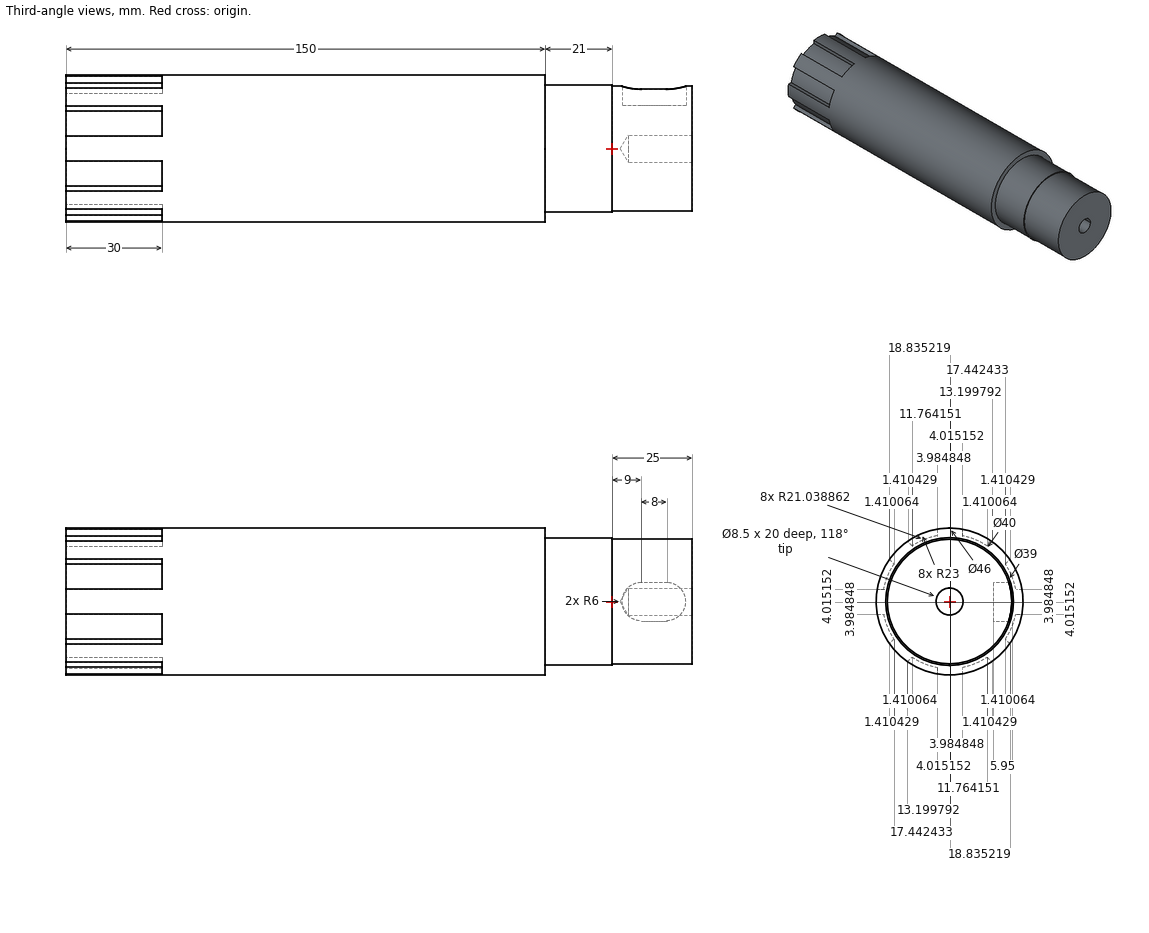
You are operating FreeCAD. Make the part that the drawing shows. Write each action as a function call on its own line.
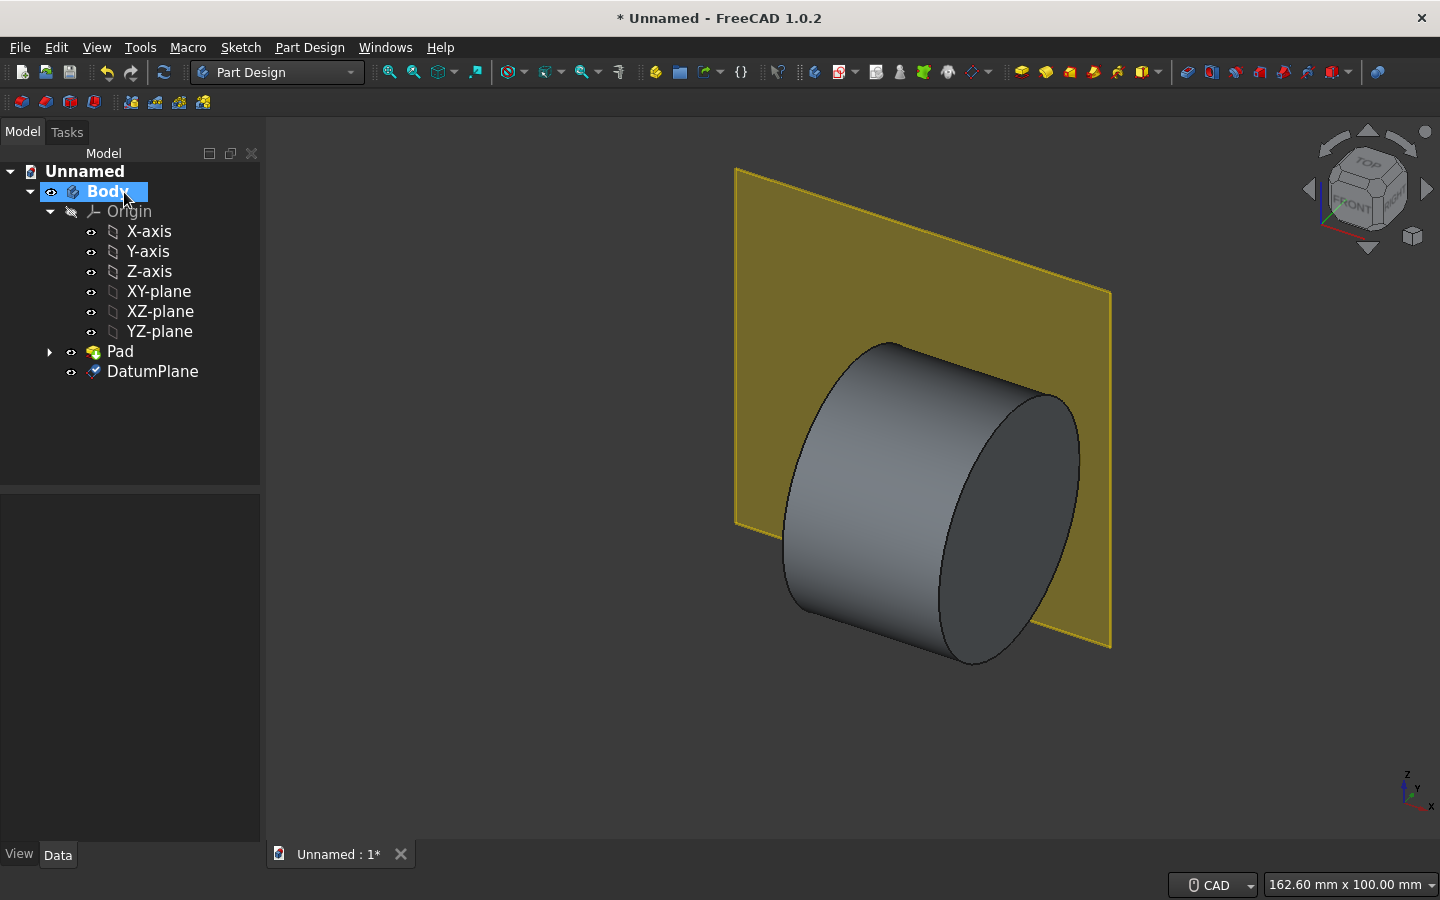
click(116, 372)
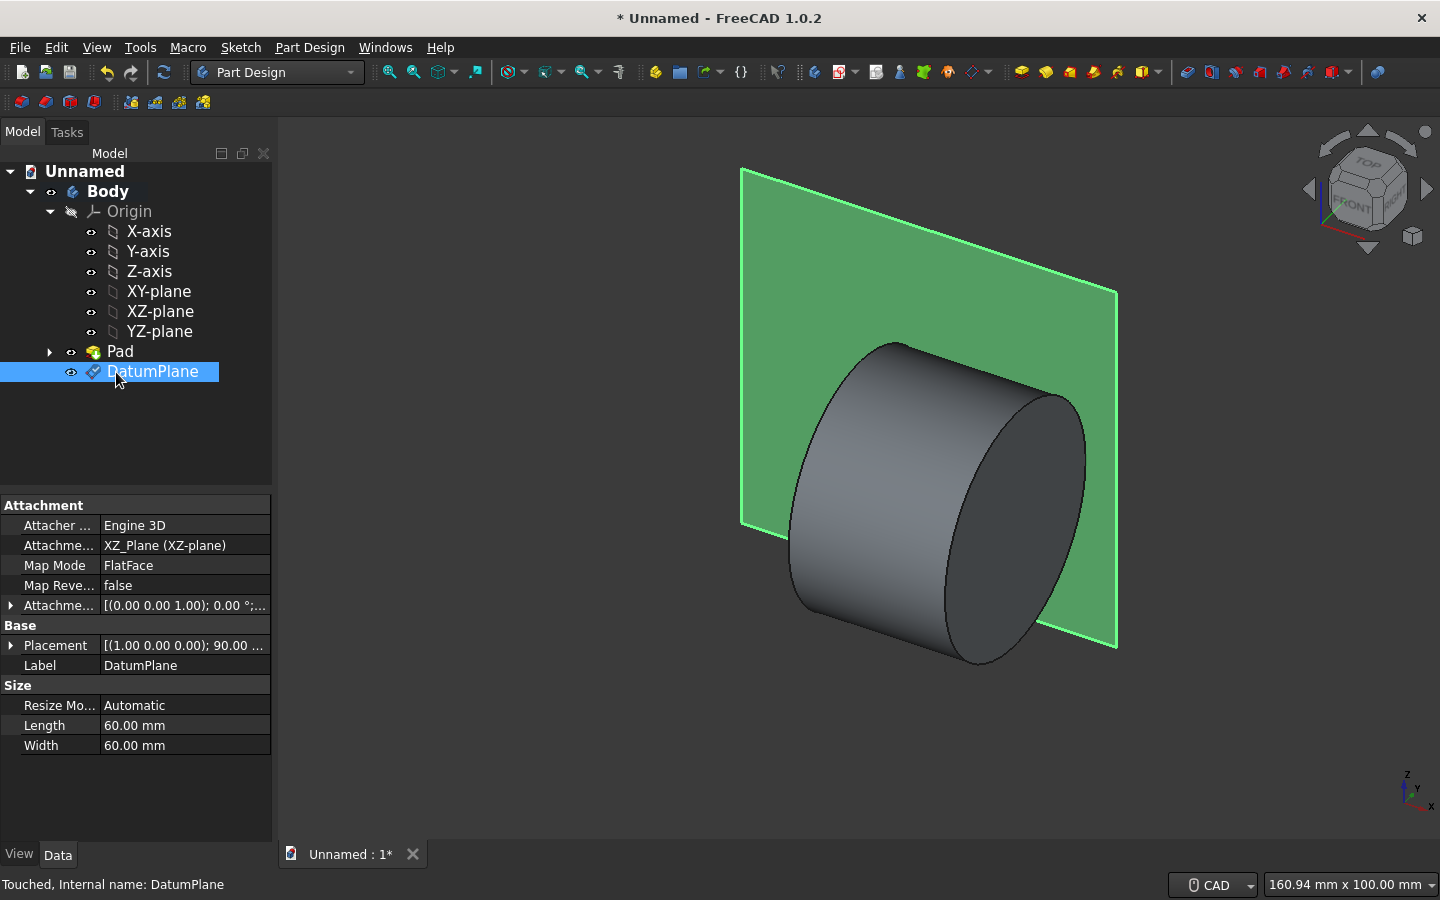
click(840, 72)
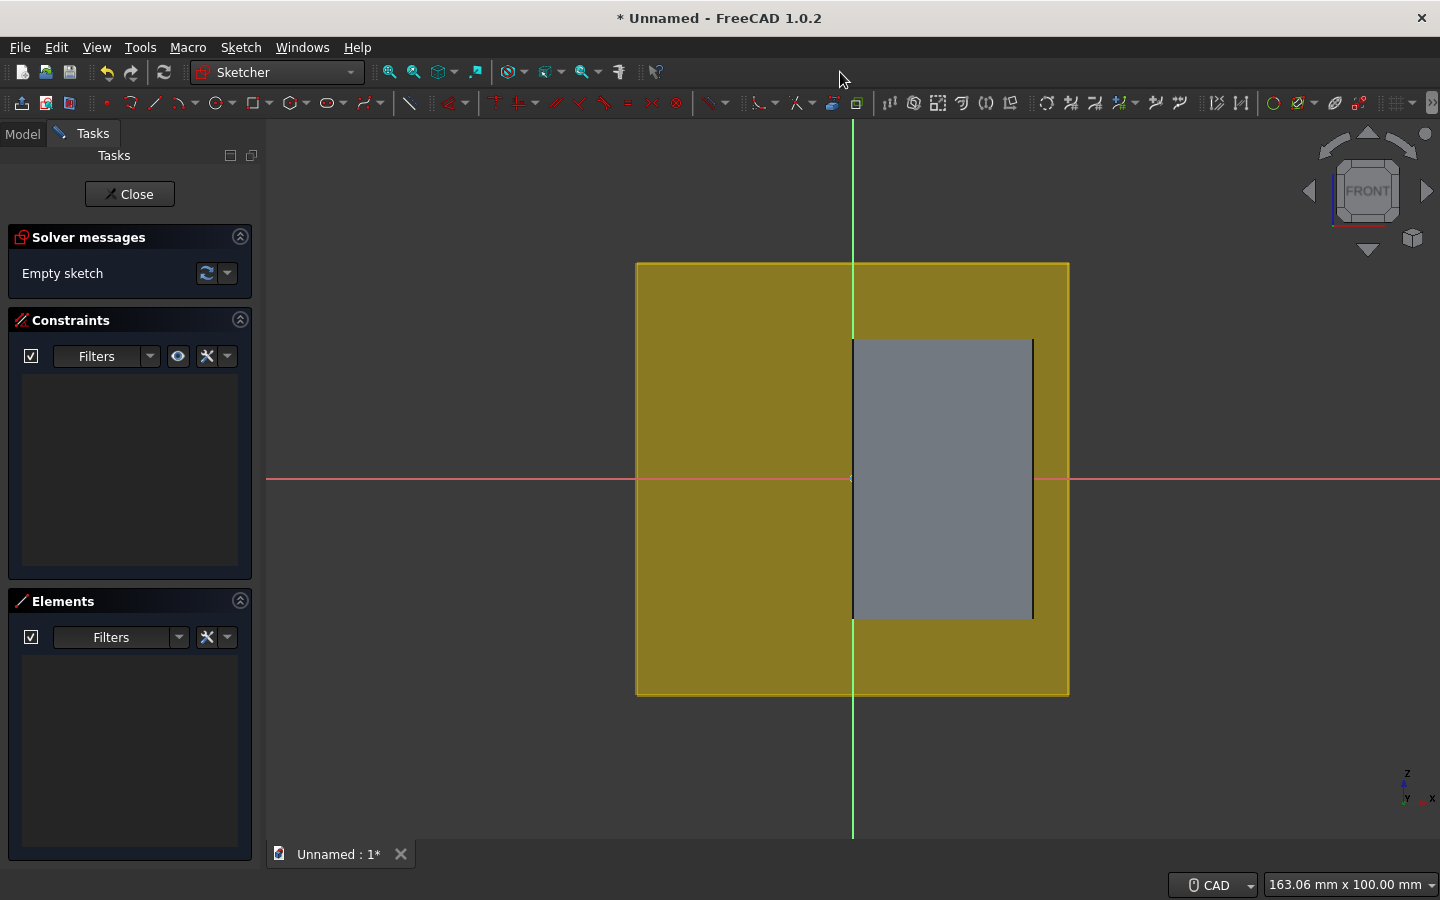
click(70, 104)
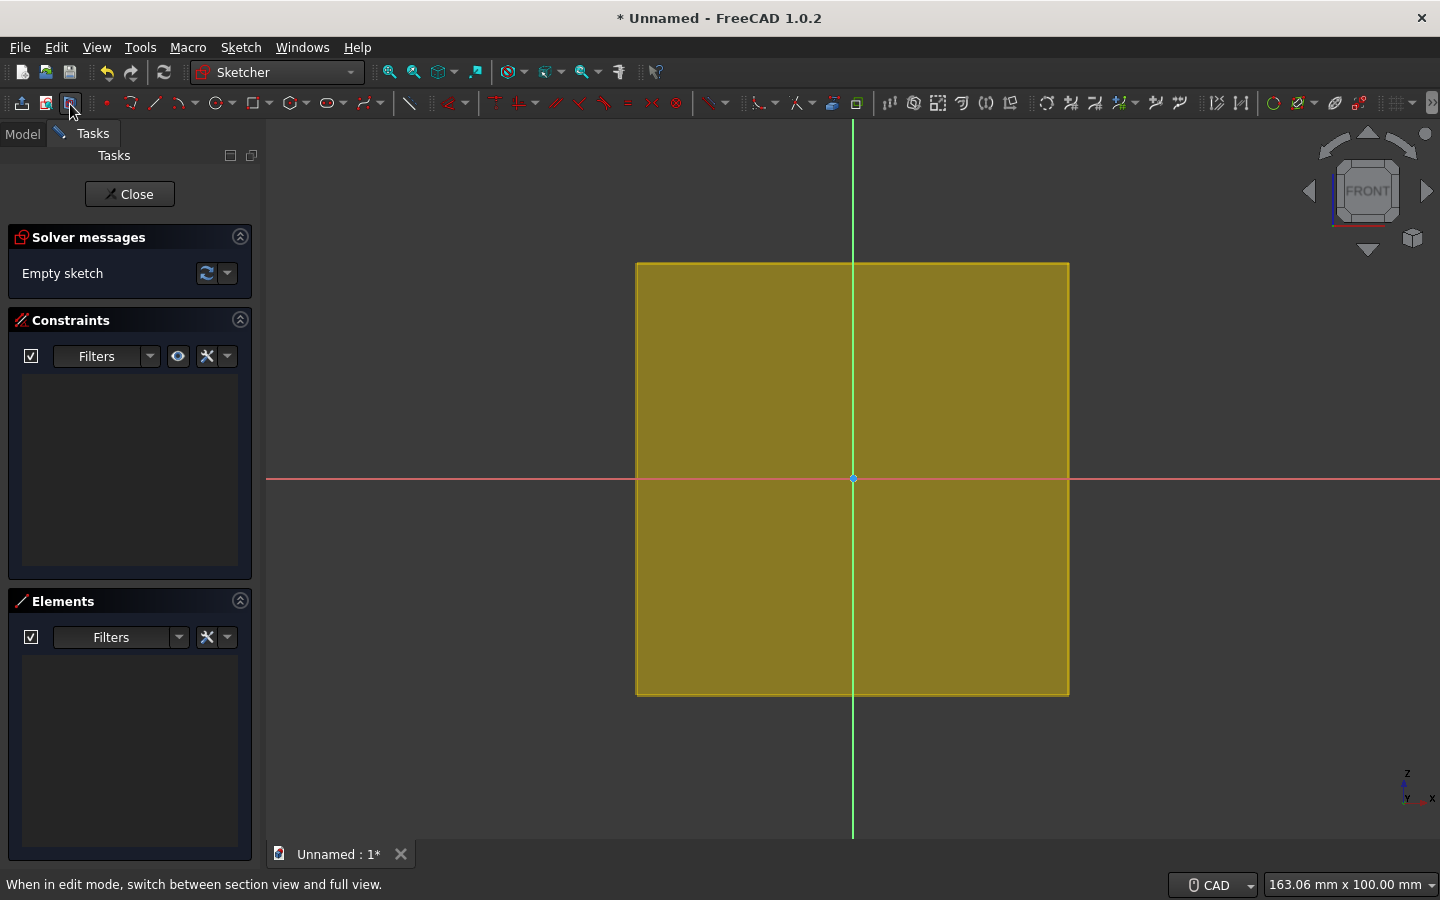
scroll(985, 479, up, 7)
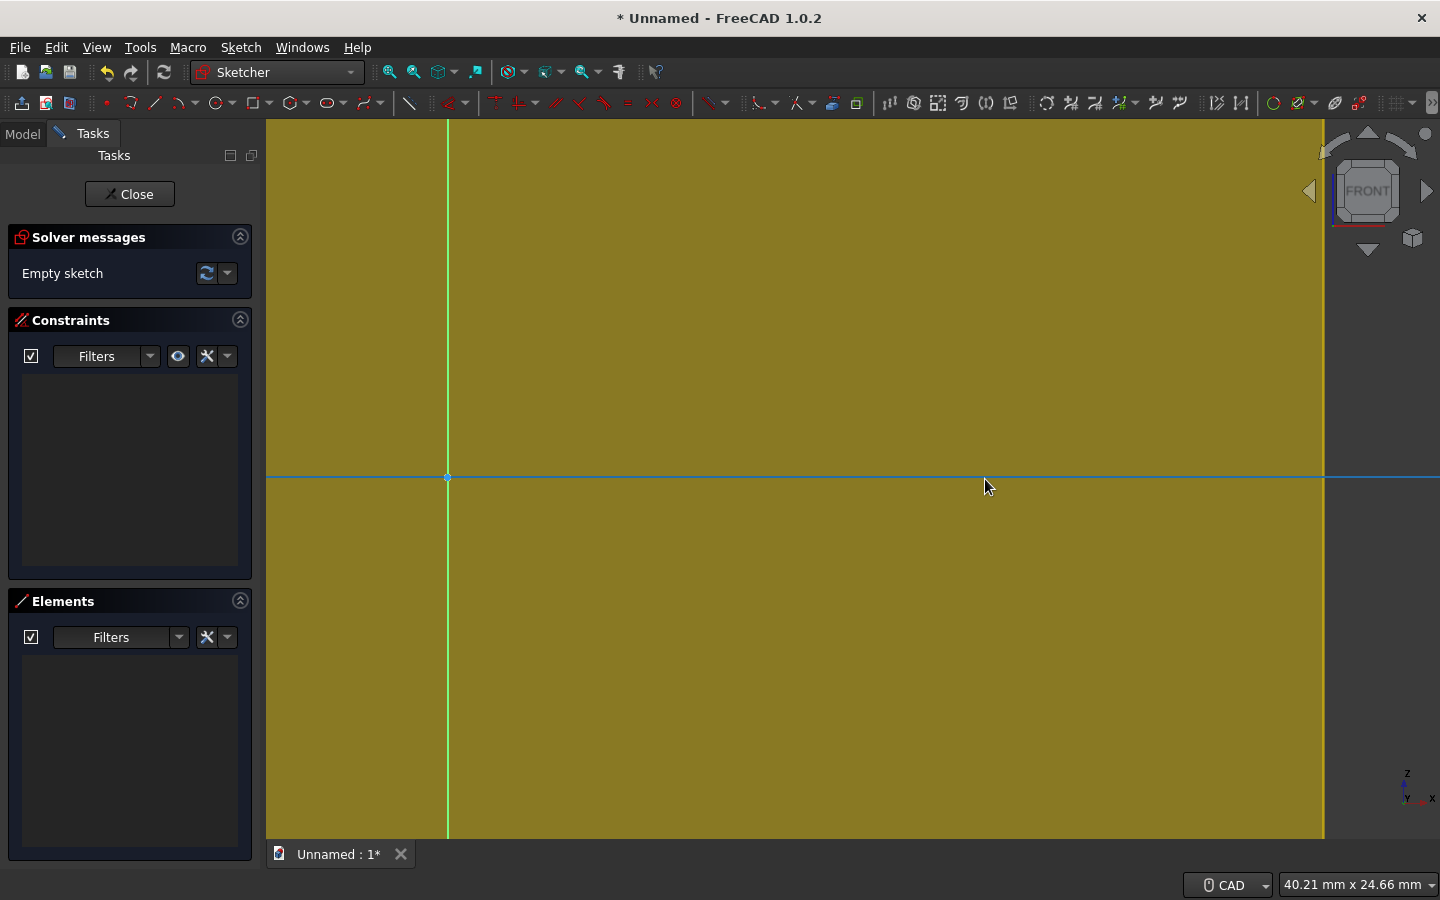
click(328, 104)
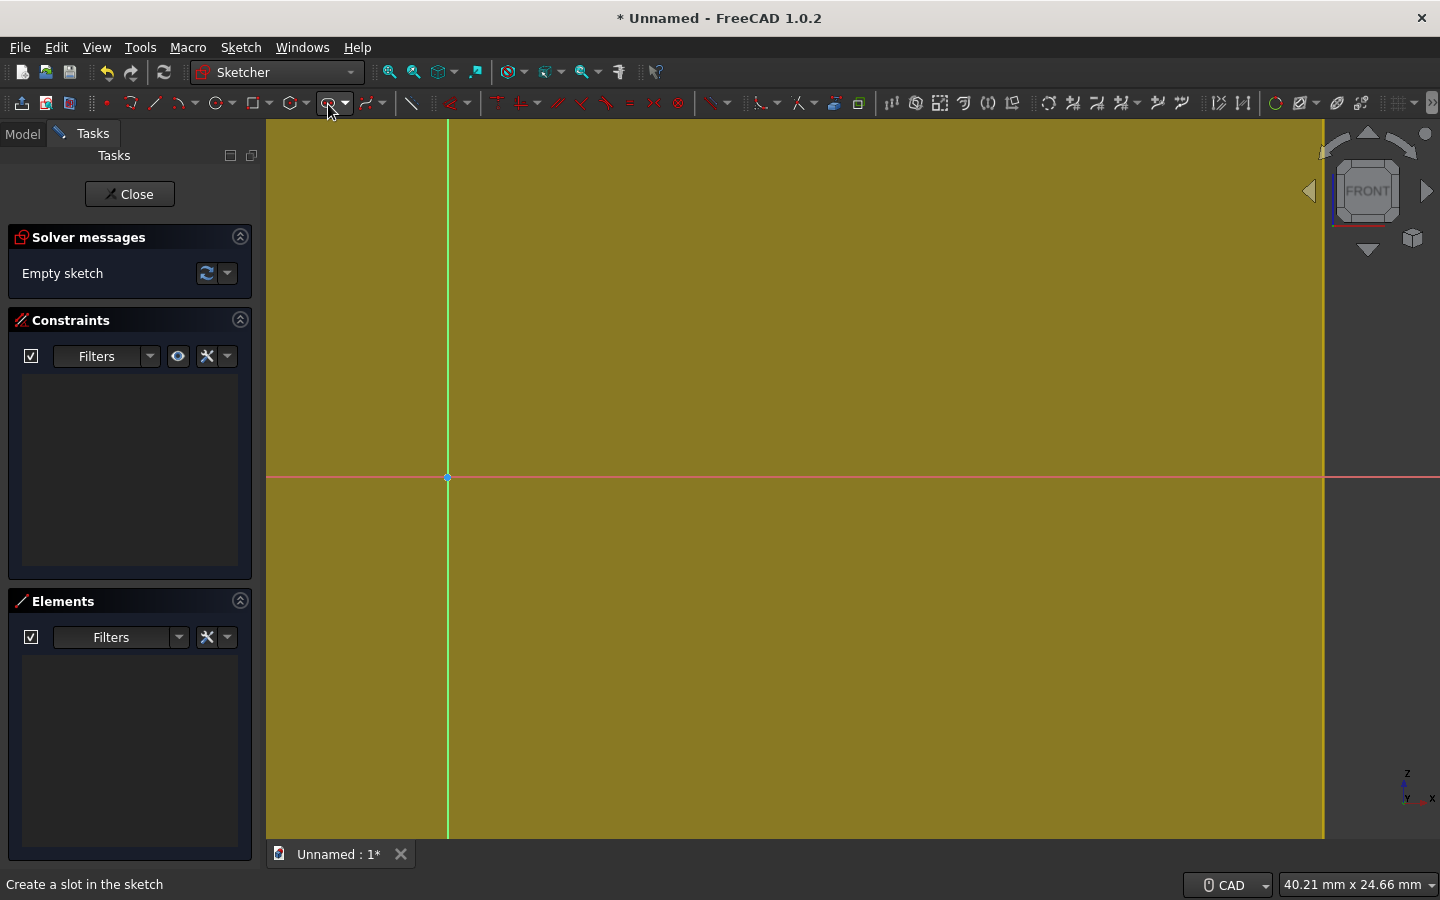
click(711, 477)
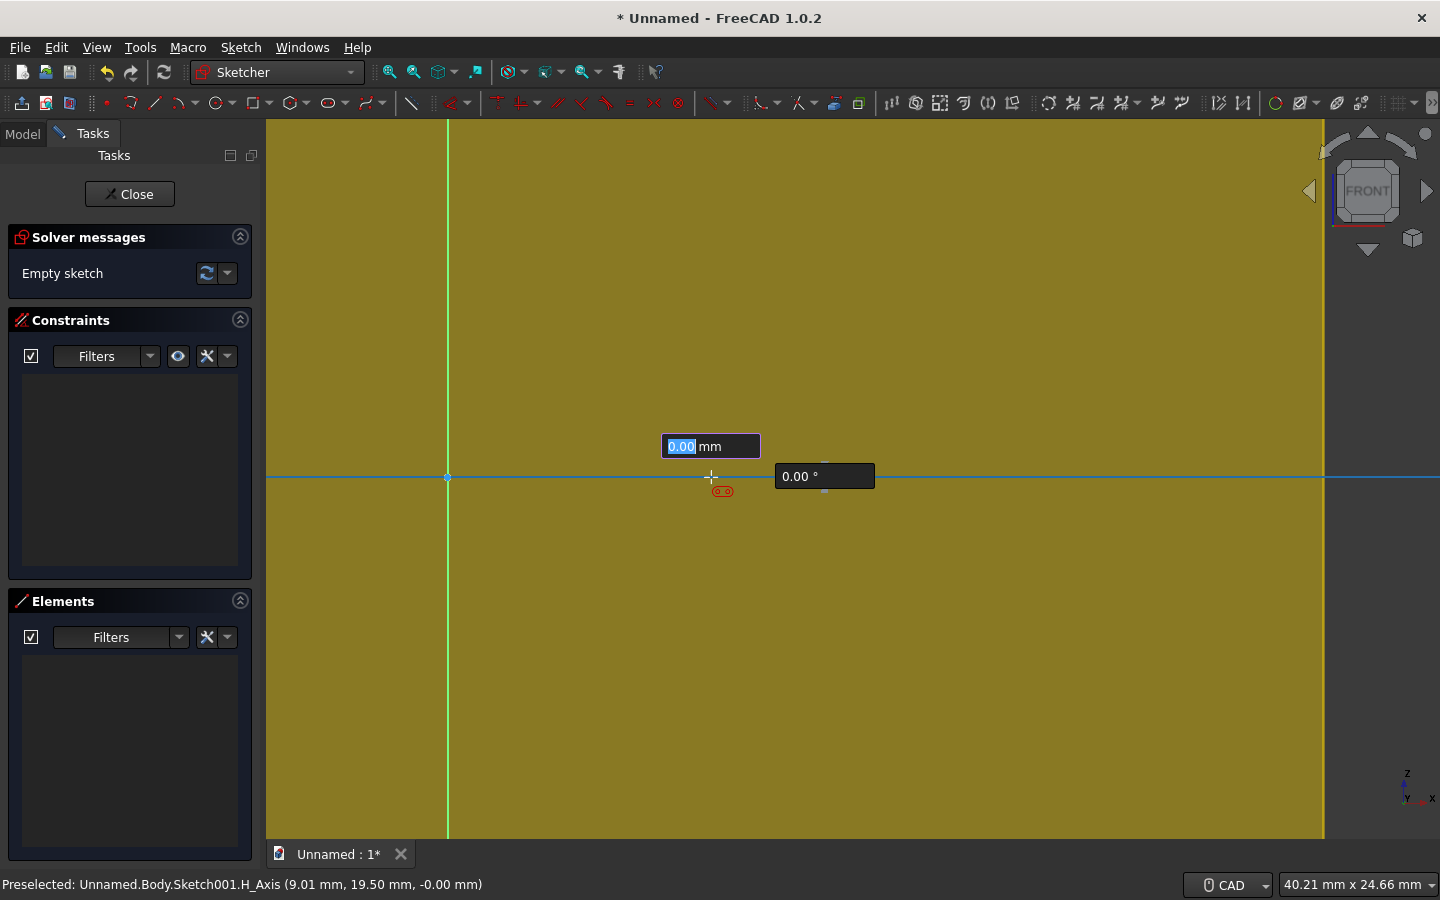
click(944, 468)